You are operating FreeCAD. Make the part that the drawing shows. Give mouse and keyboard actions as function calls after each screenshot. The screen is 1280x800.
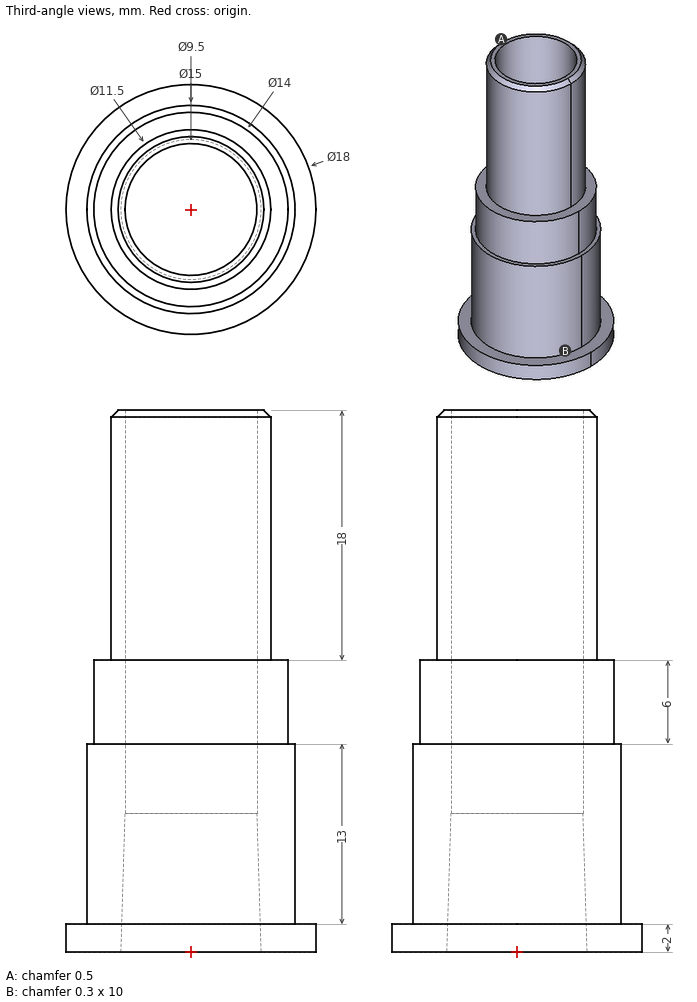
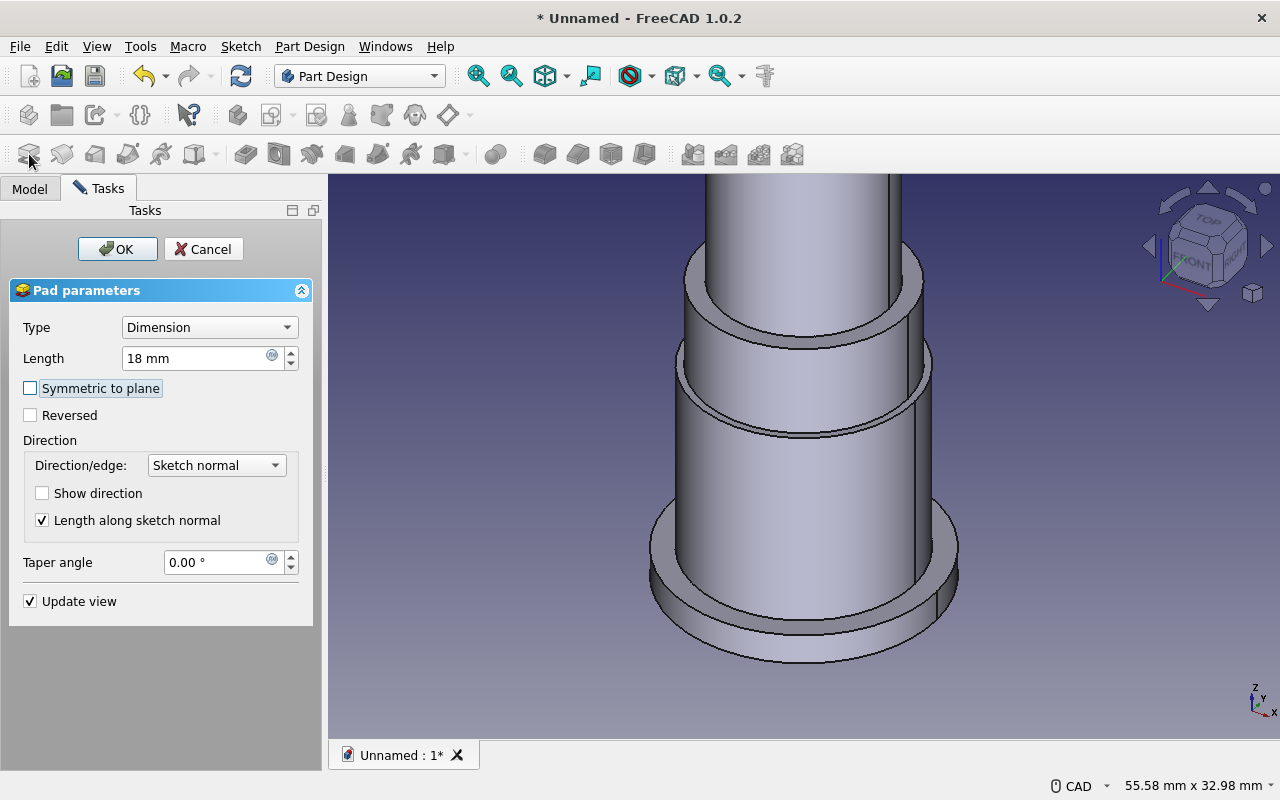
click(118, 249)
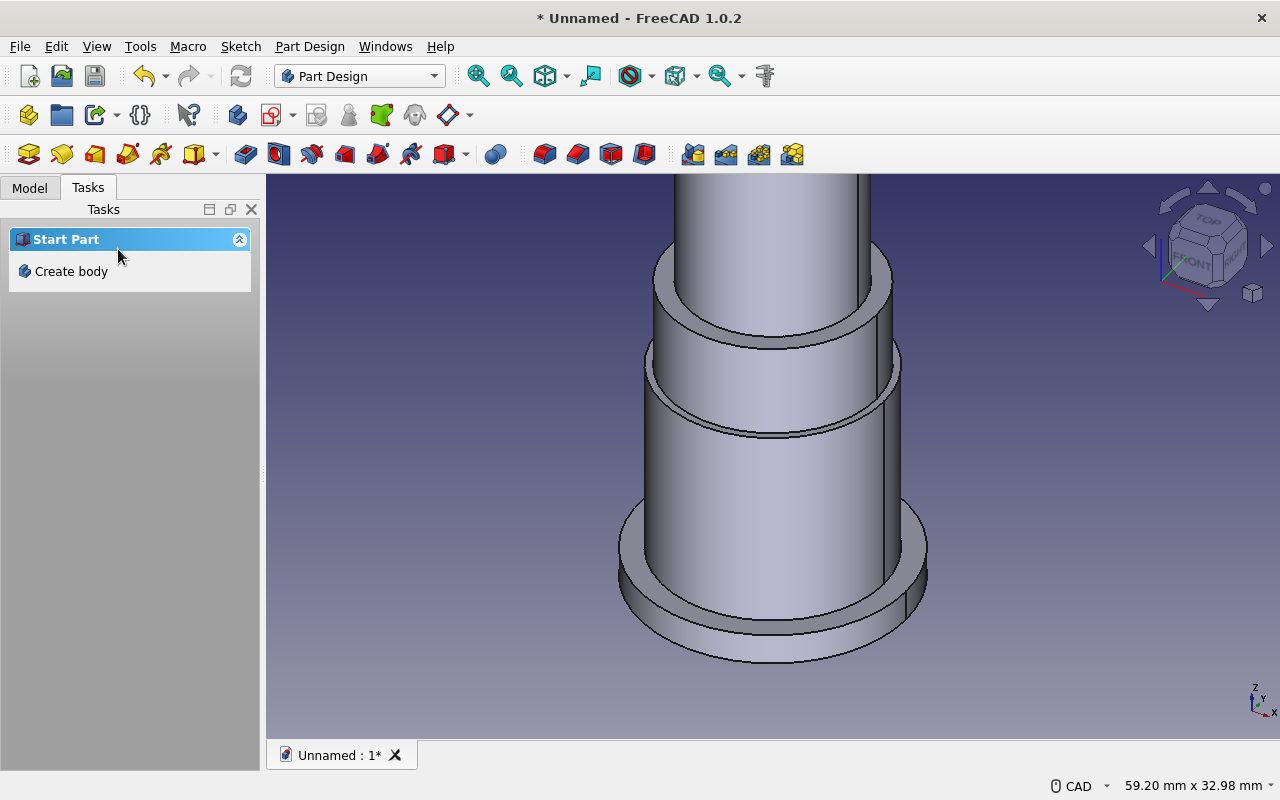
click(479, 76)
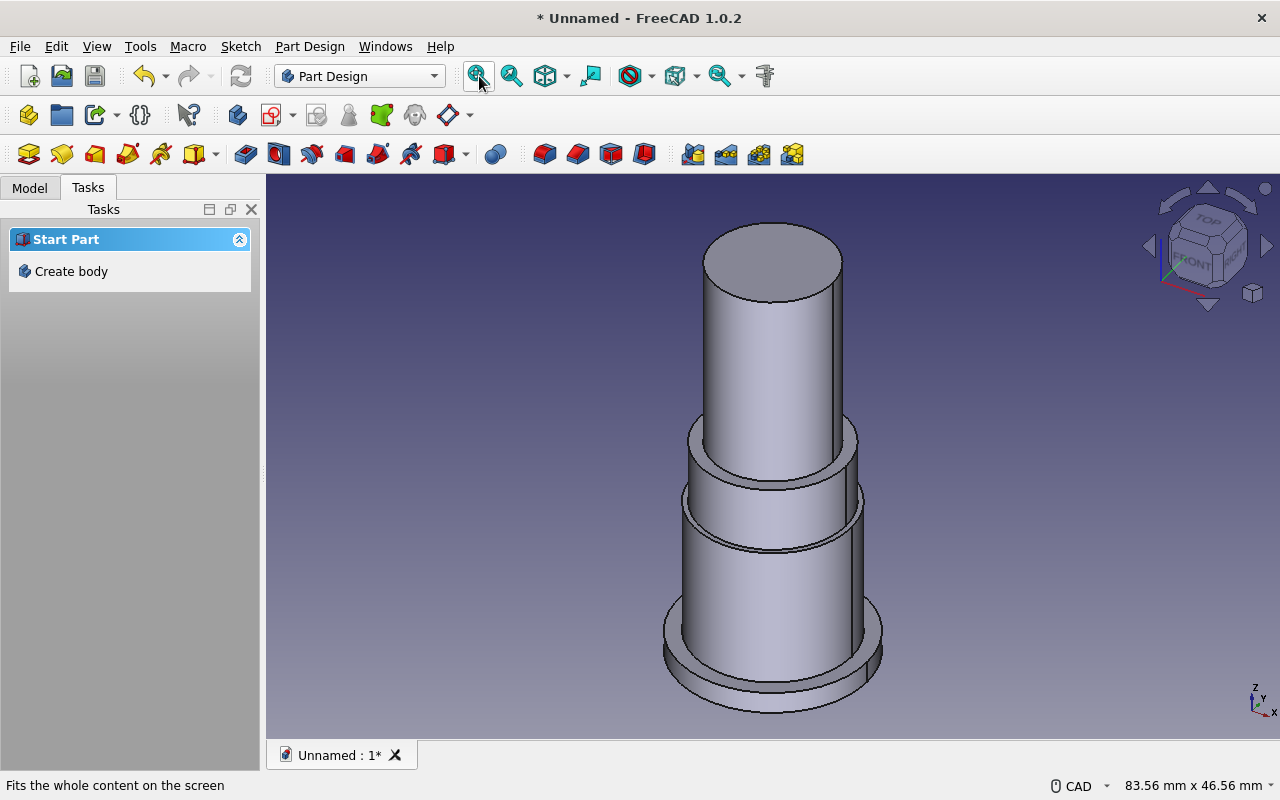
click(270, 116)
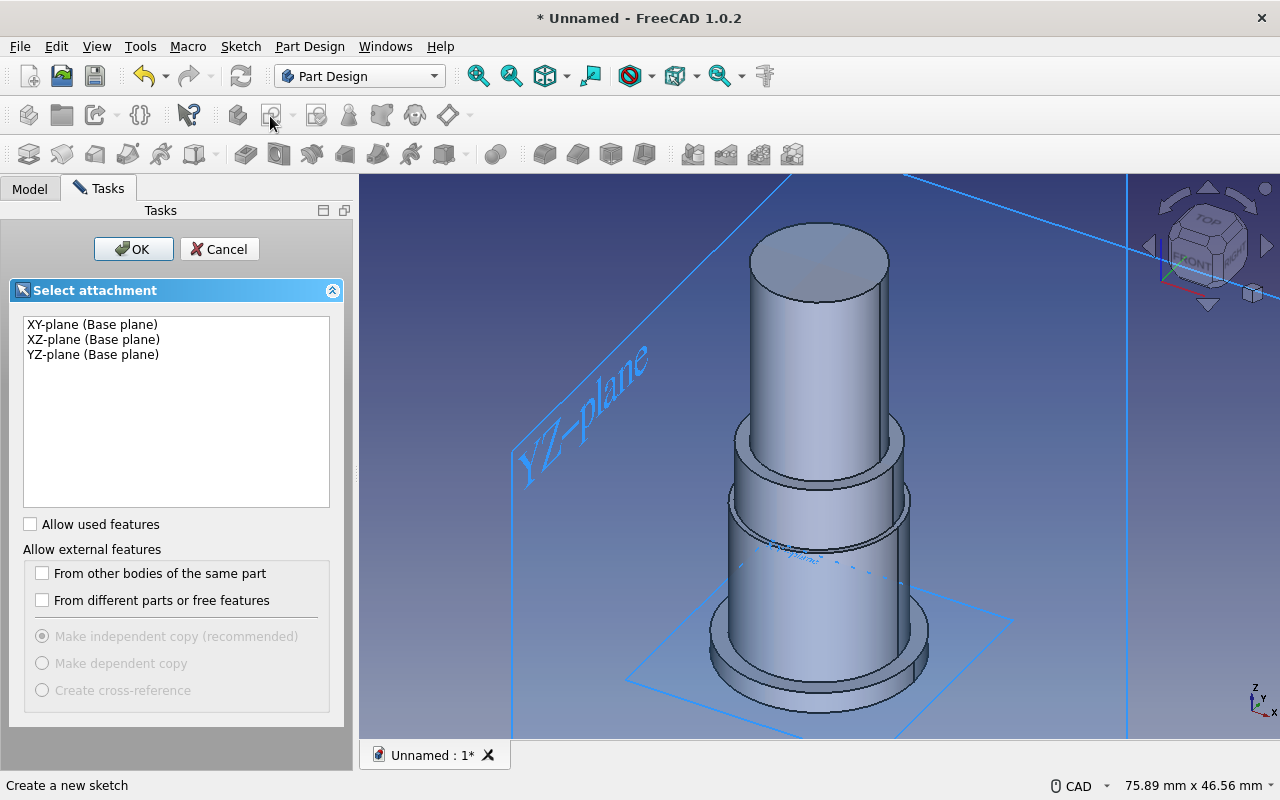
click(84, 324)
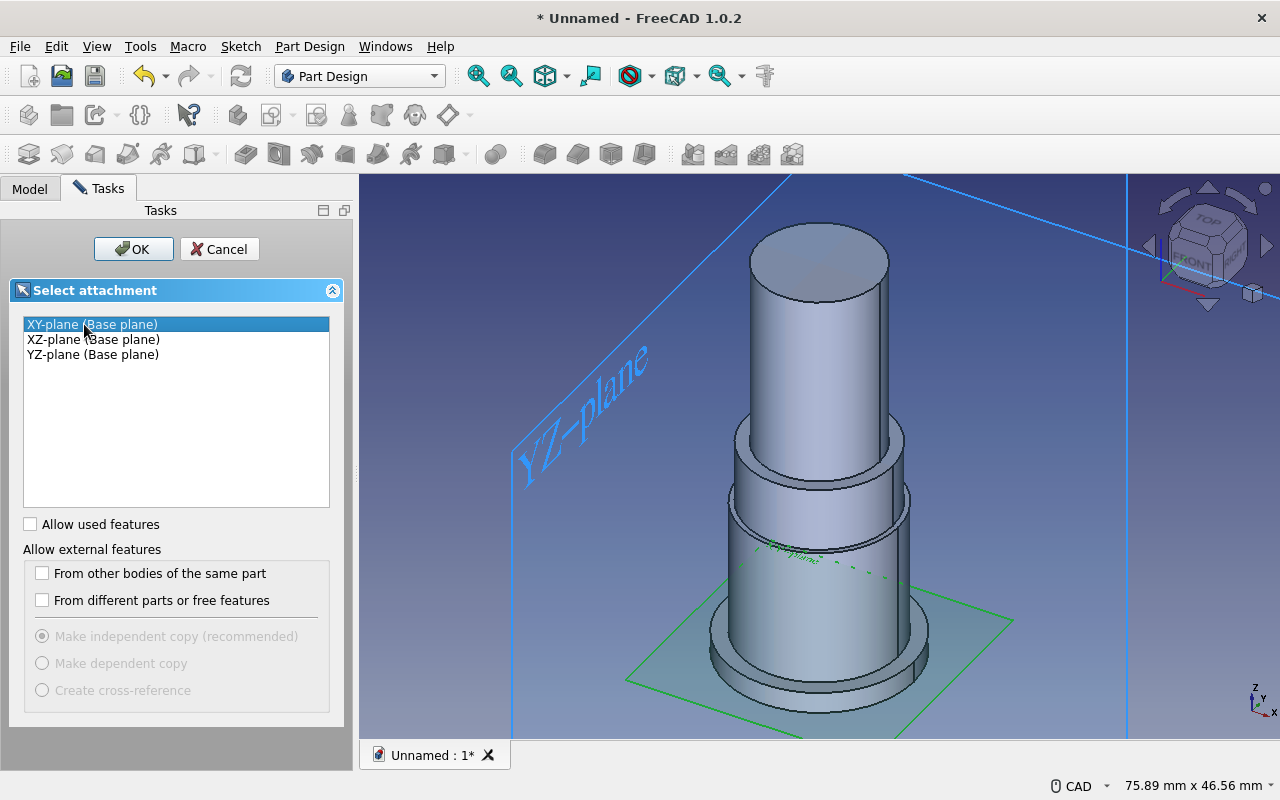
click(134, 249)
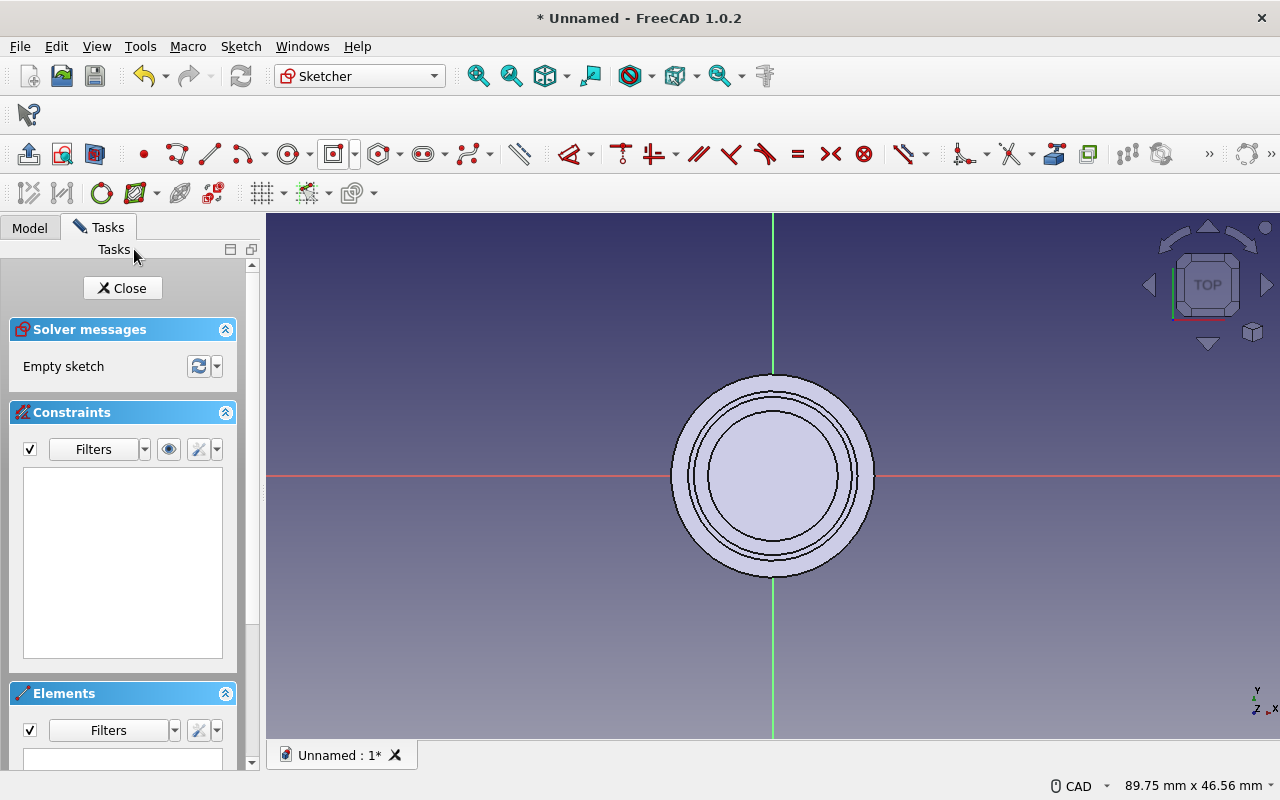
click(95, 154)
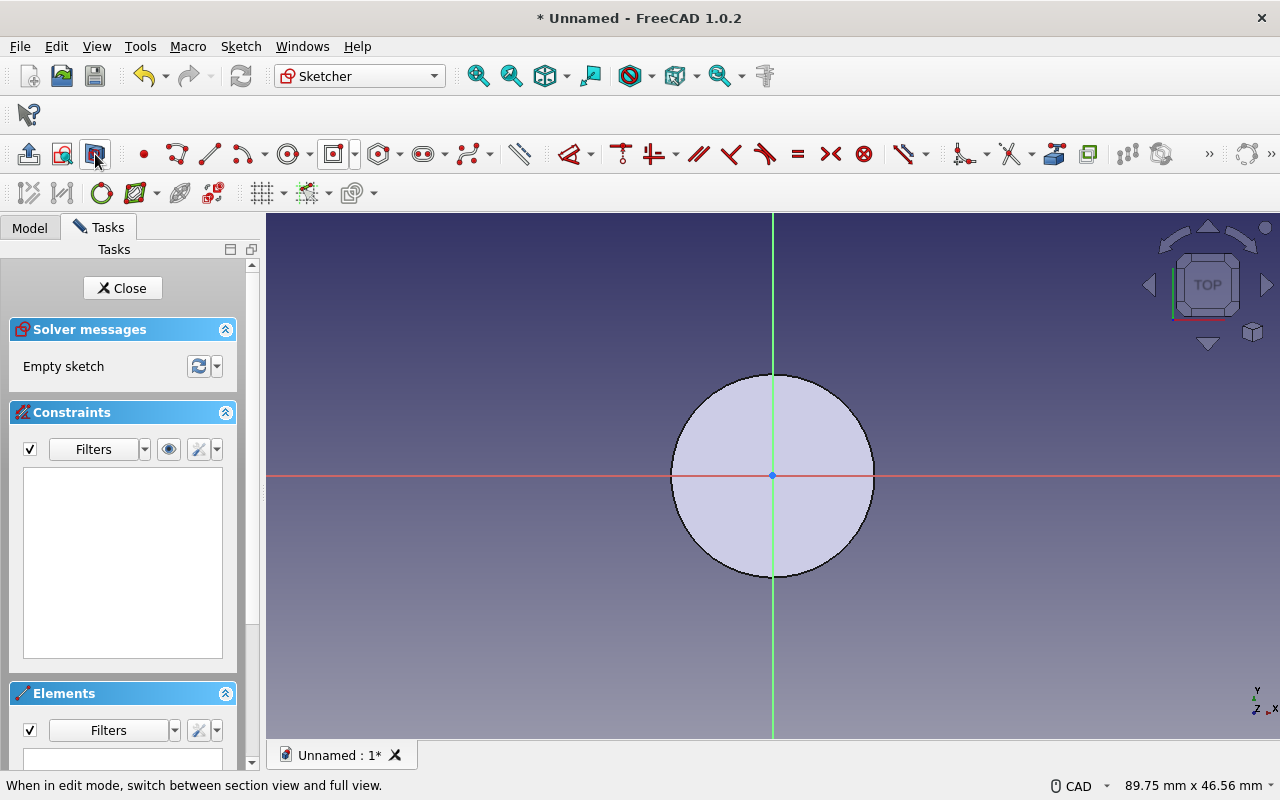
scroll(802, 476, up, 6)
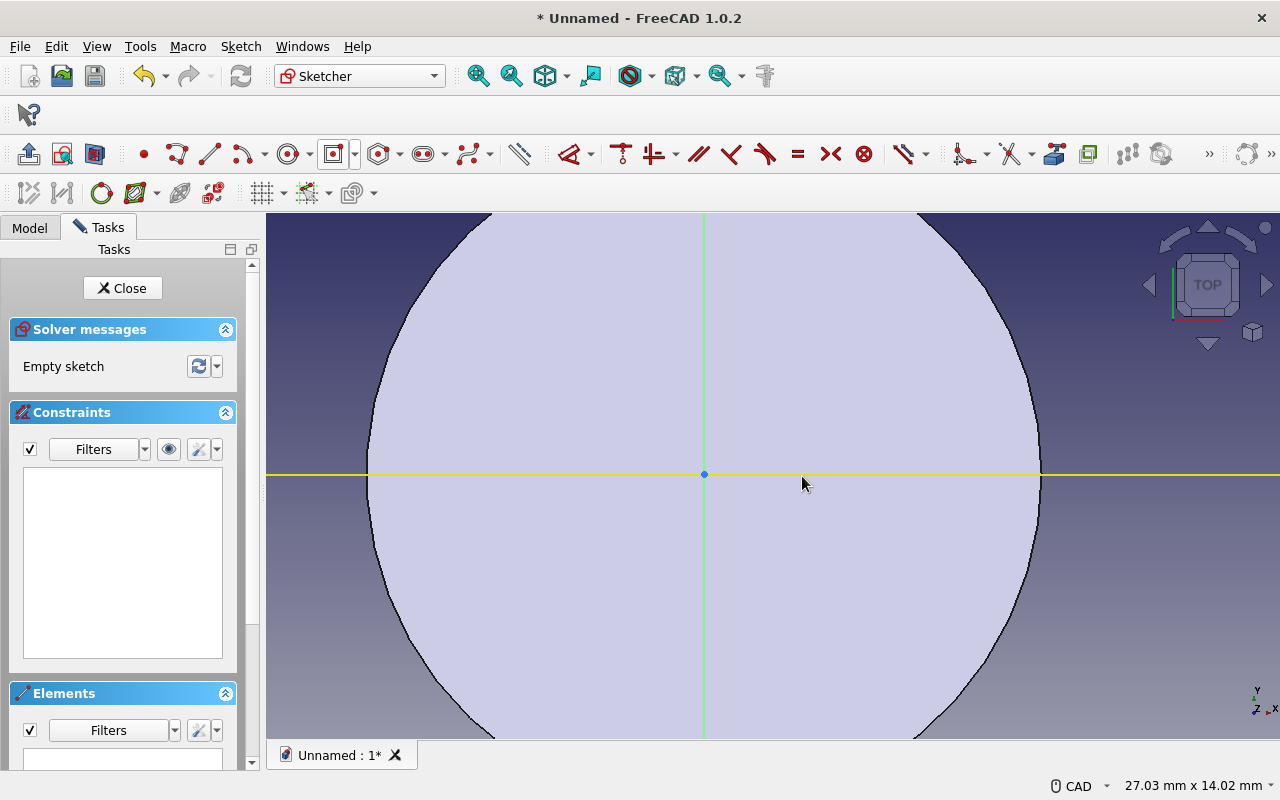
click(288, 154)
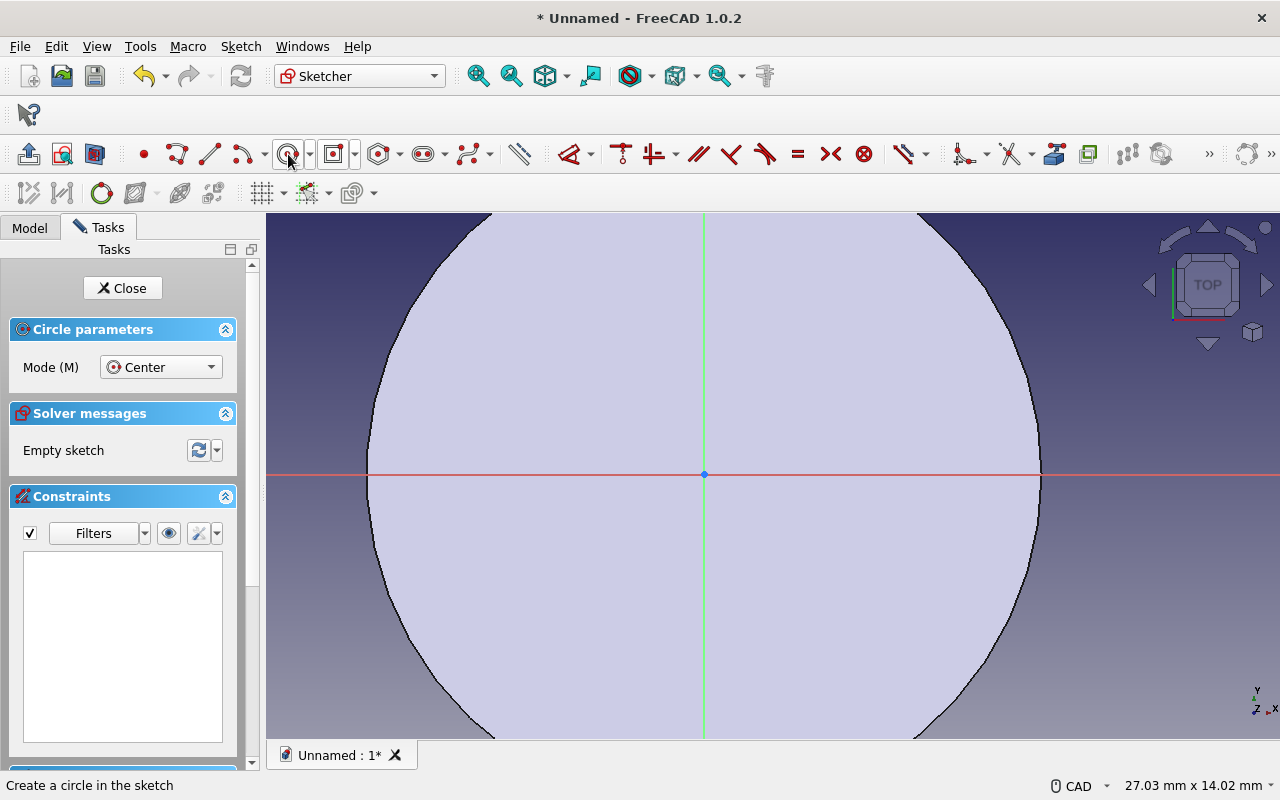
click(704, 475)
click(830, 349)
key(Escape)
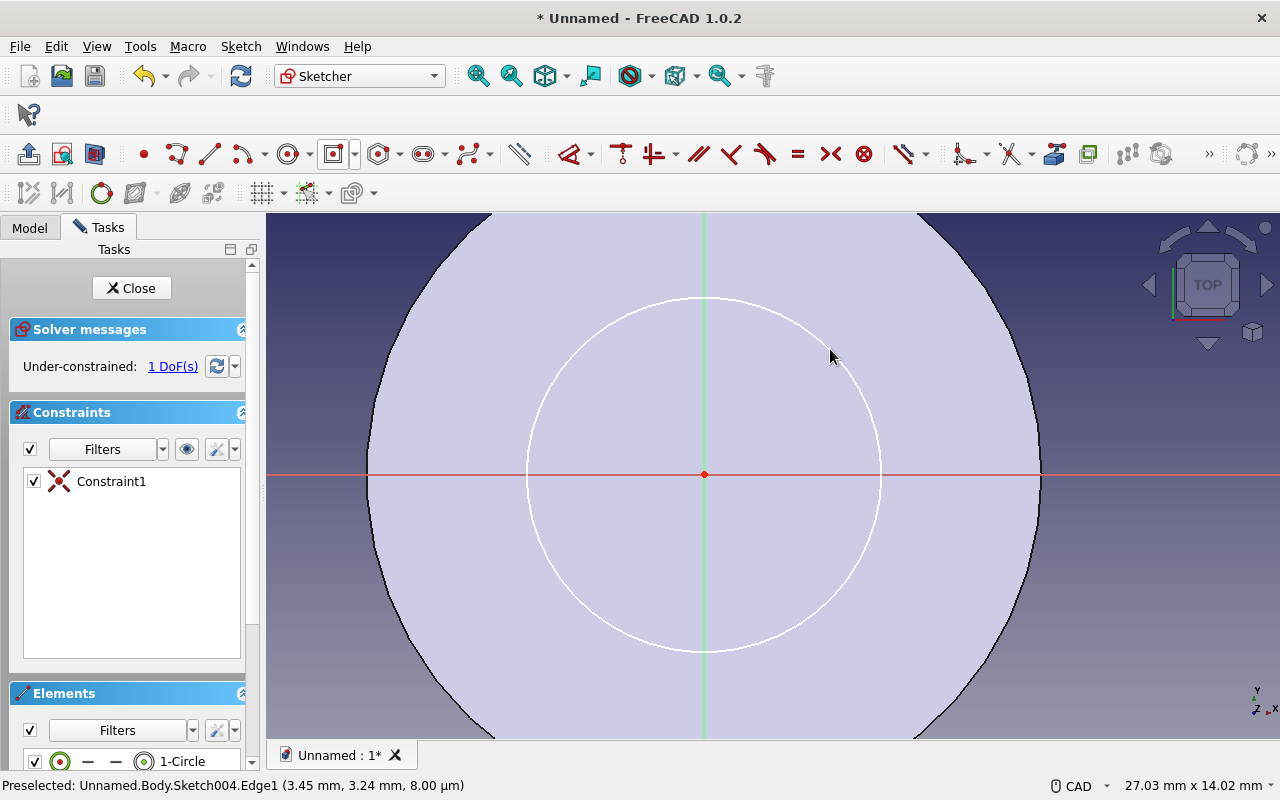
click(568, 154)